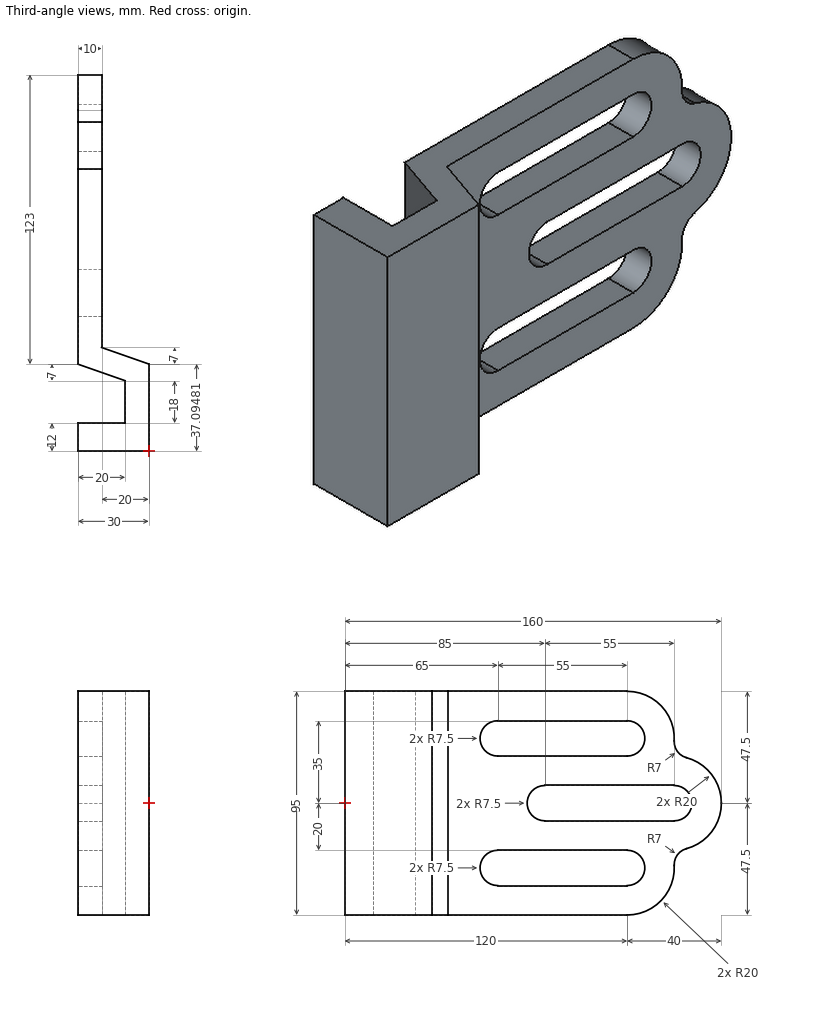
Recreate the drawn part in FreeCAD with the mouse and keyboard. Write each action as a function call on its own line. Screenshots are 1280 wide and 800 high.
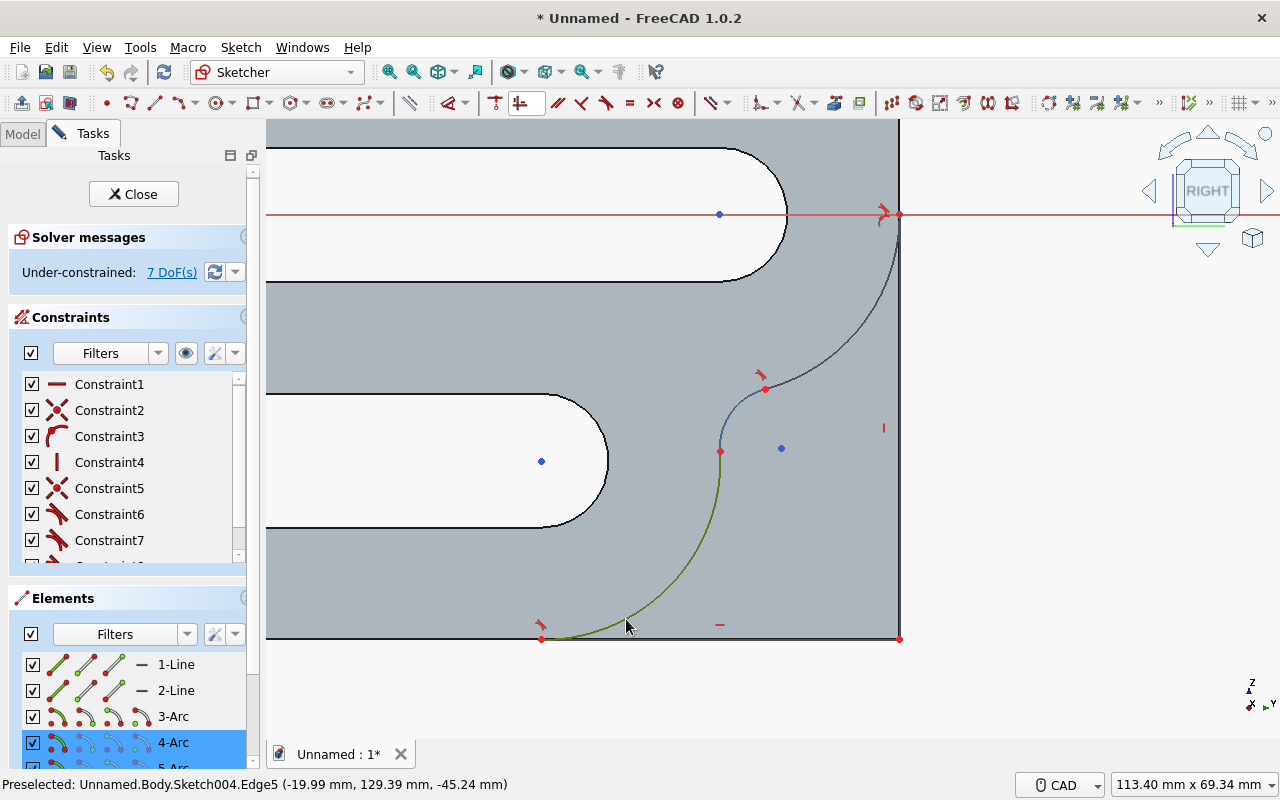
click(606, 104)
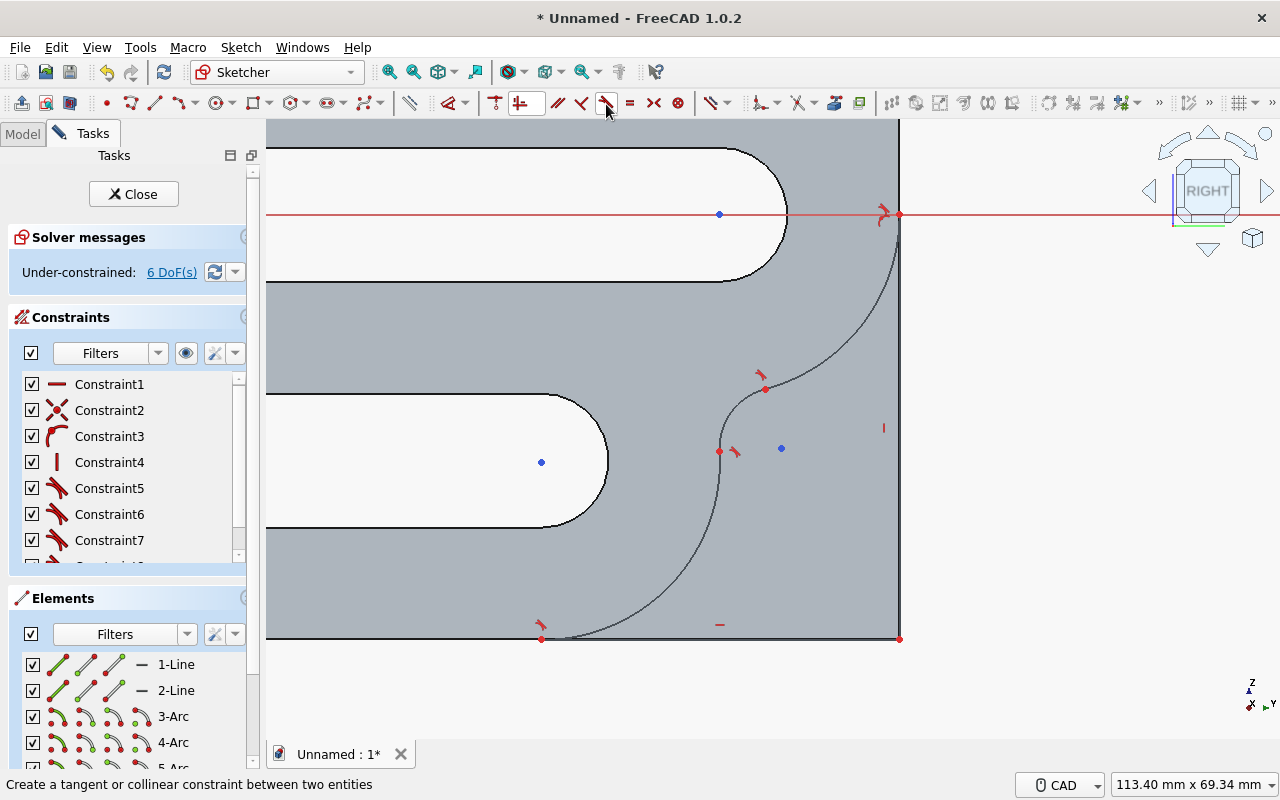
click(829, 358)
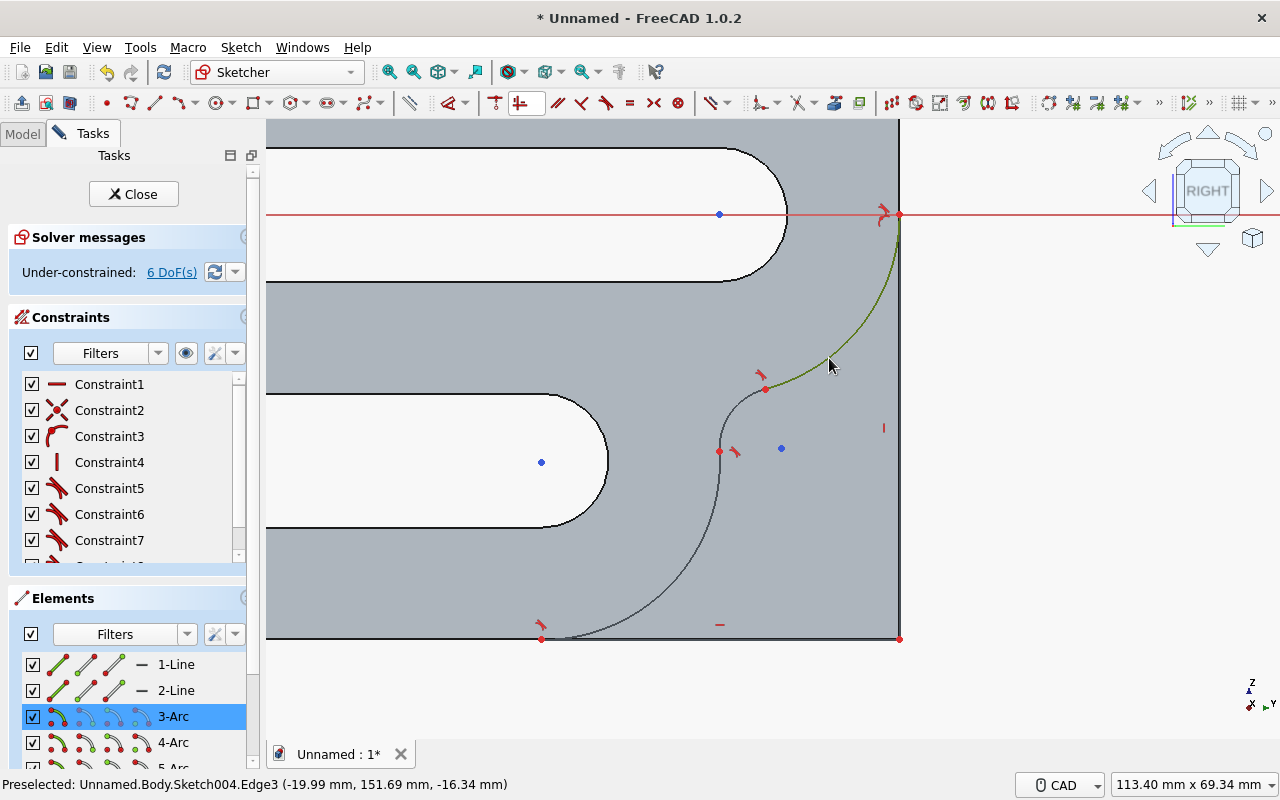
click(625, 619)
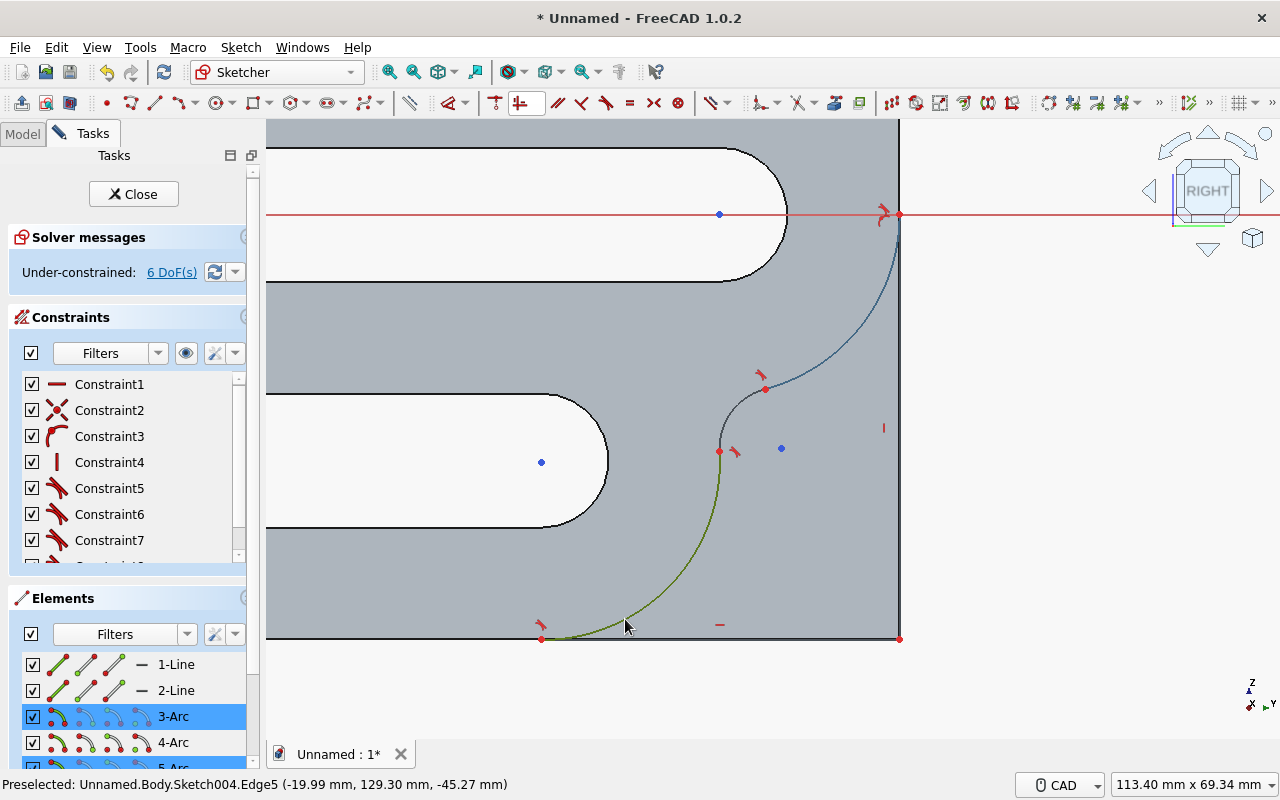
click(630, 104)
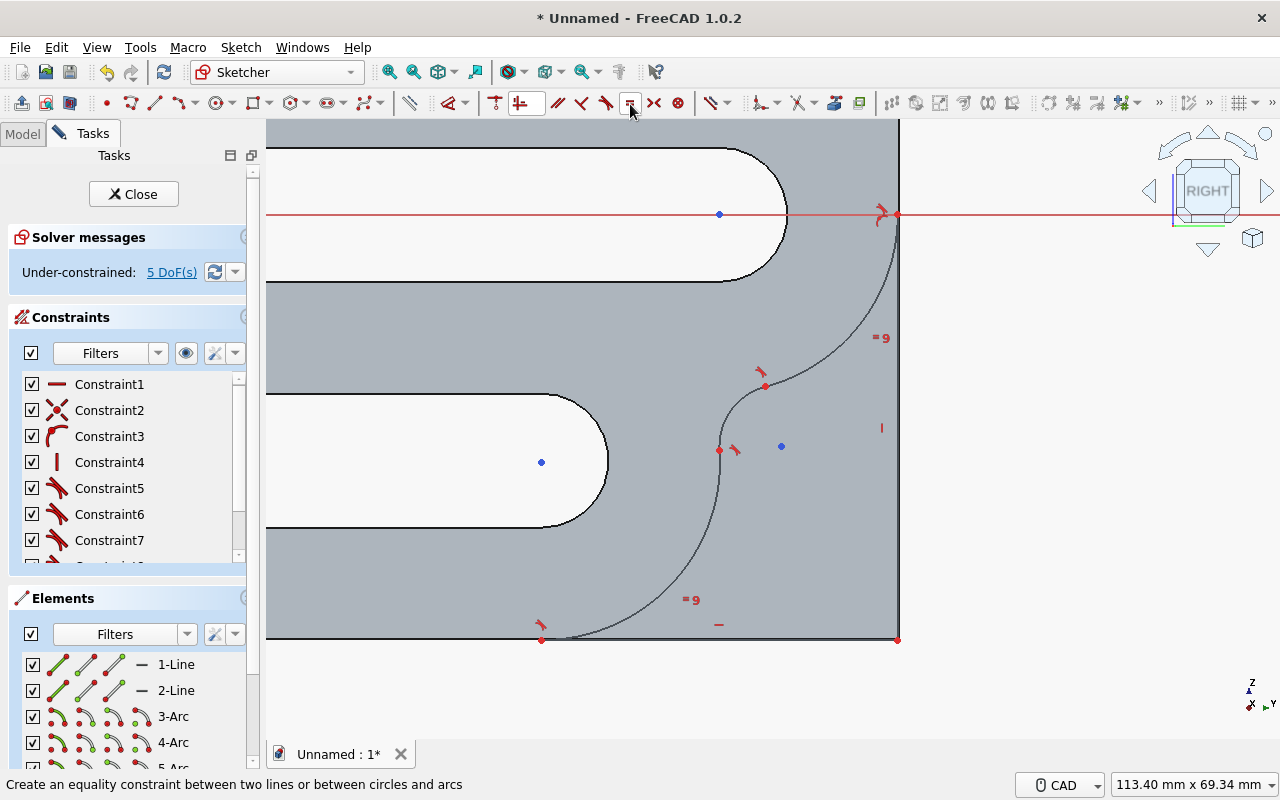
click(448, 104)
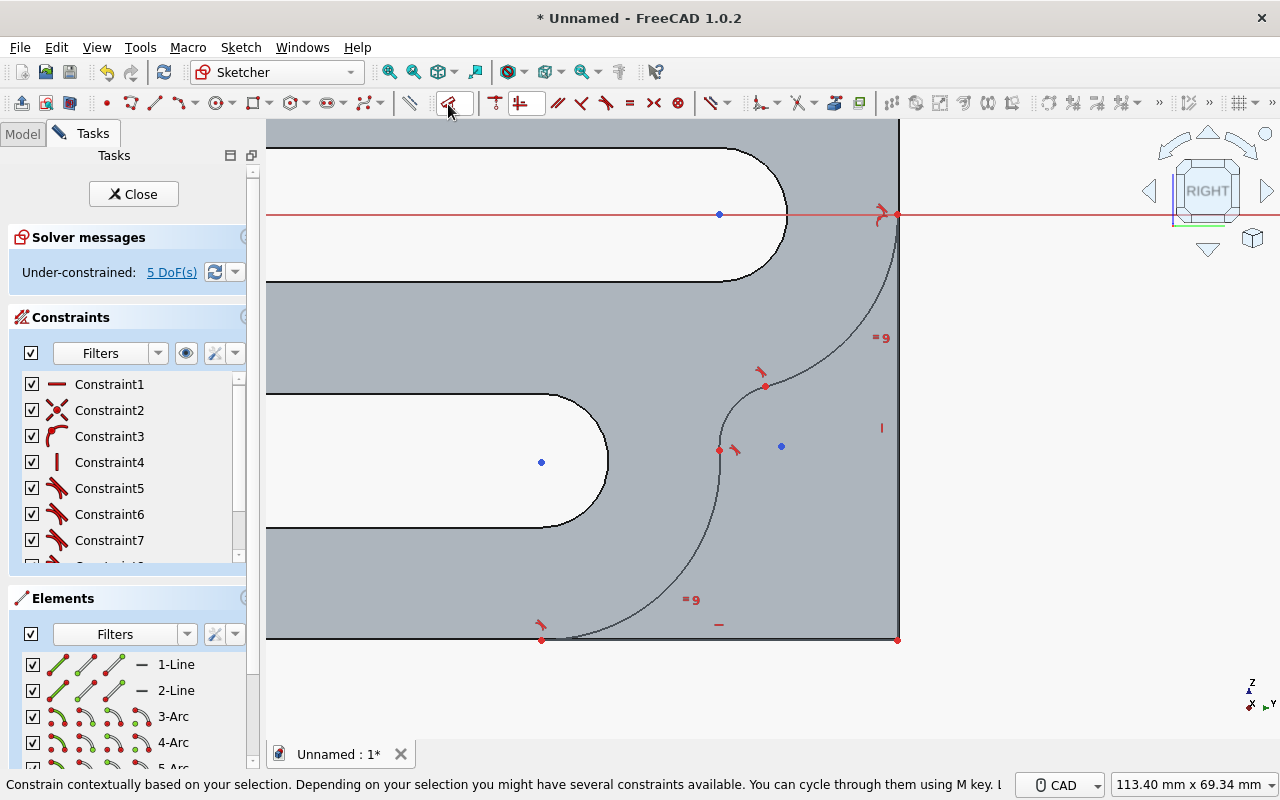
click(828, 356)
click(847, 381)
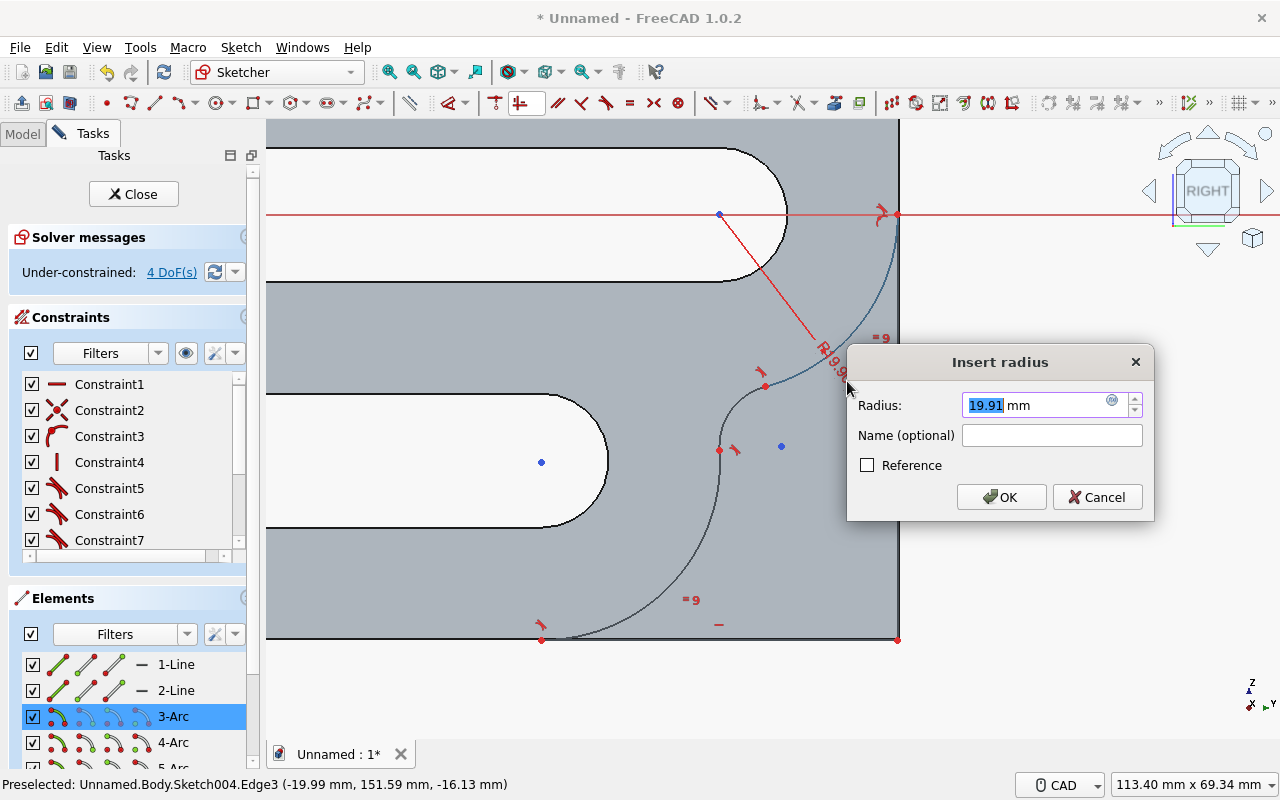
text(20)
key(Return)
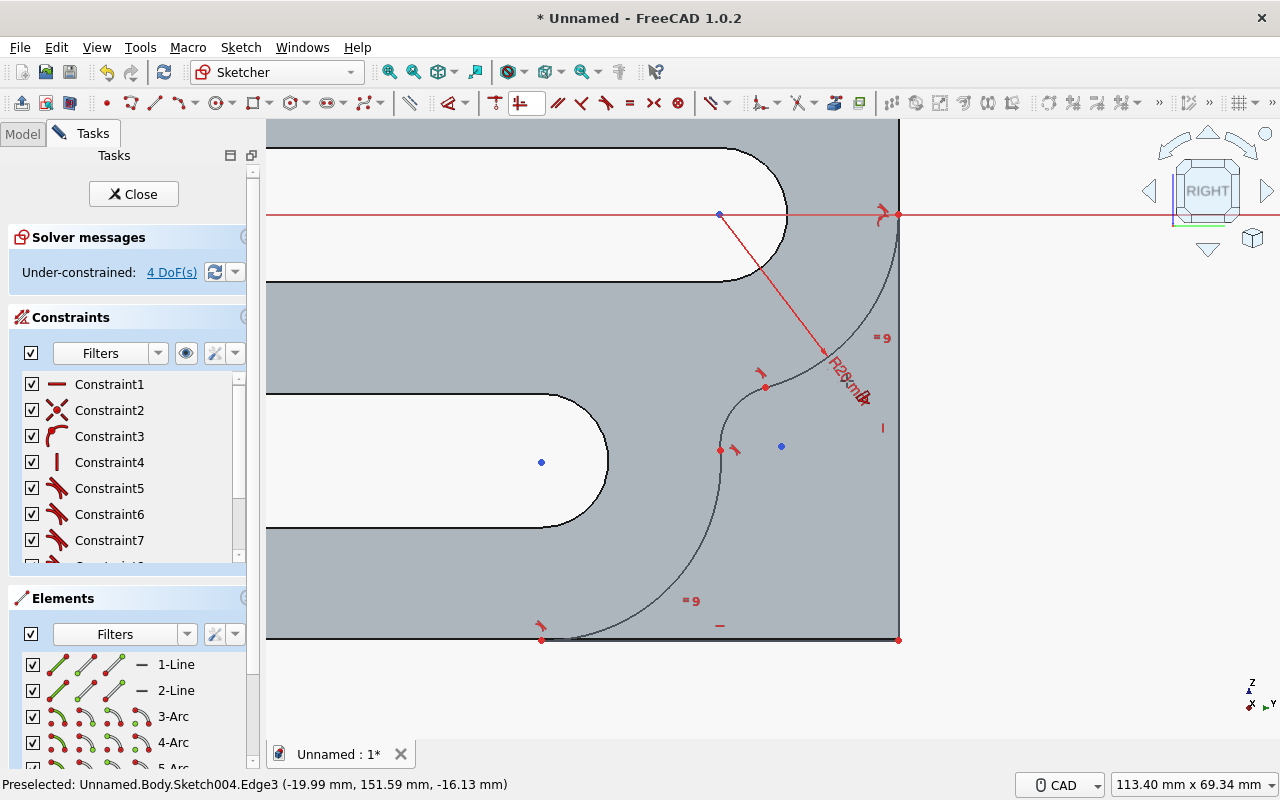
click(743, 399)
click(723, 374)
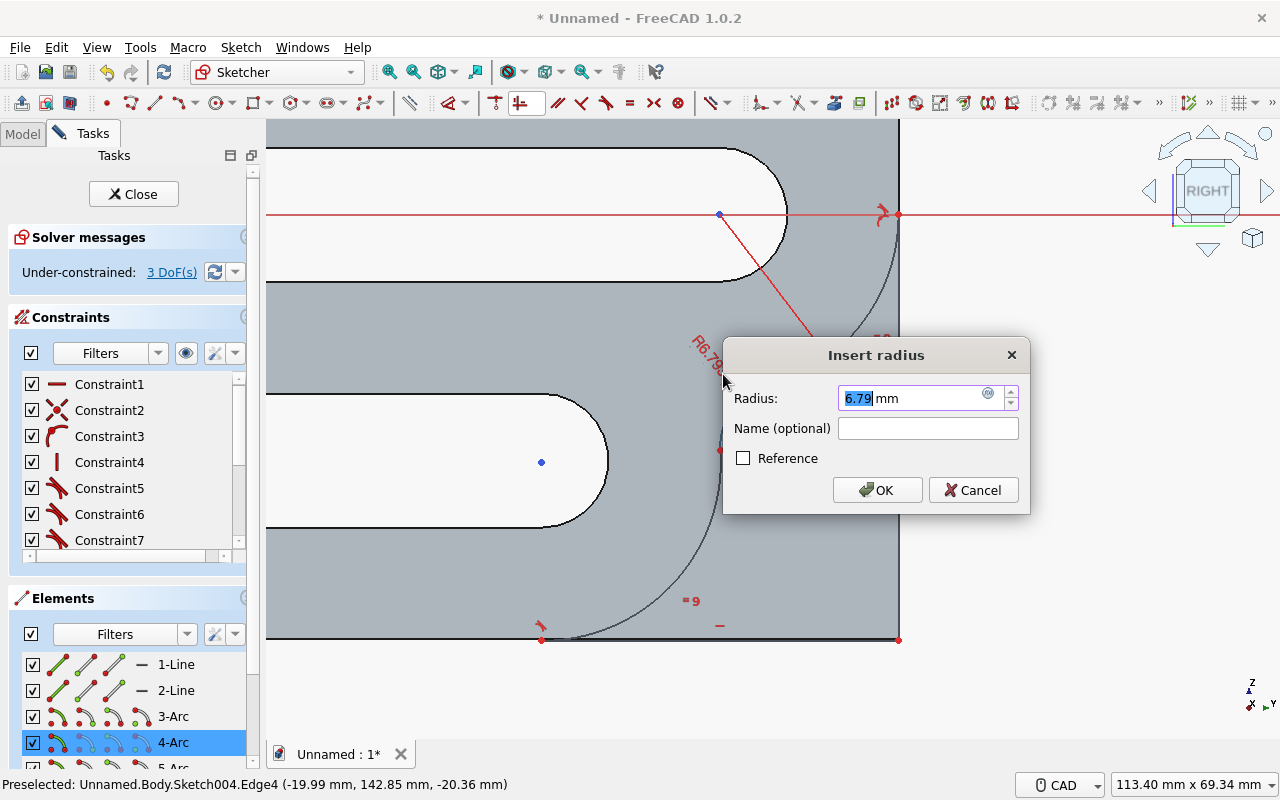
text(7)
key(Return)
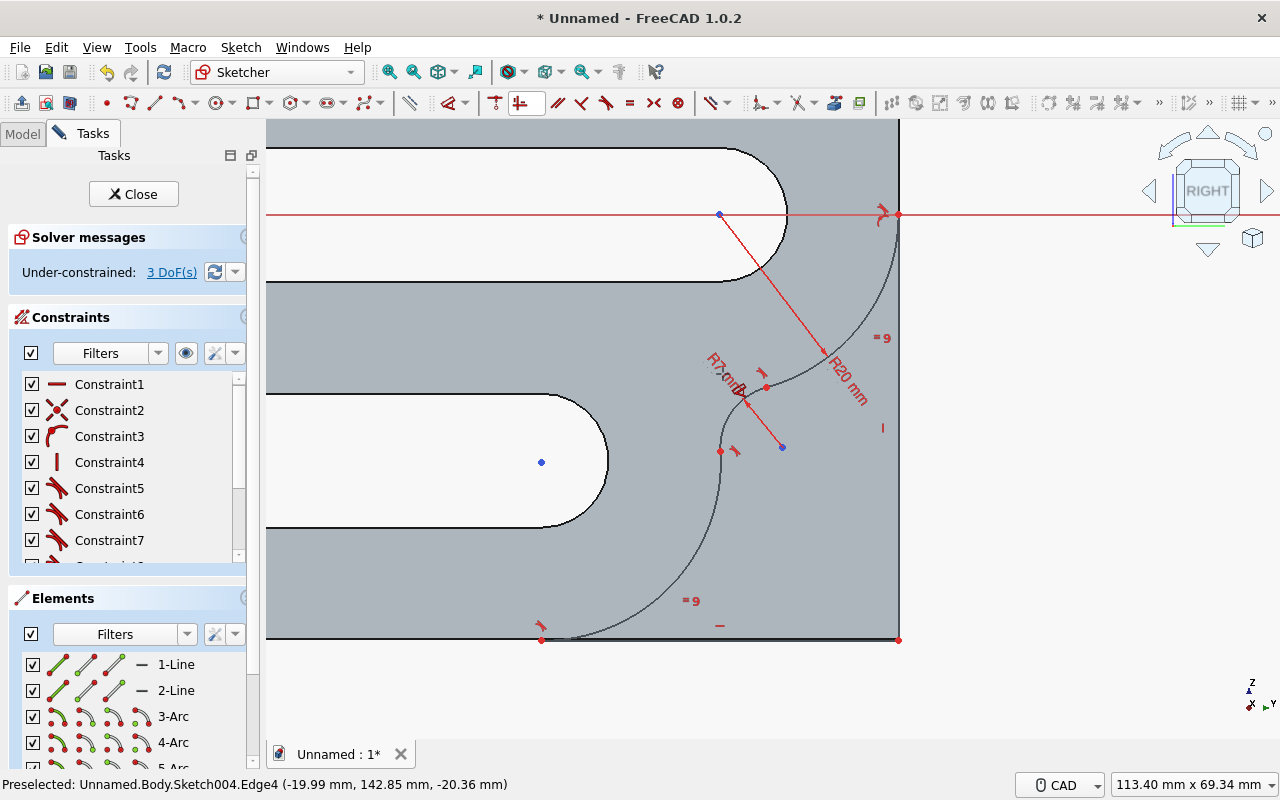
click(649, 641)
click(720, 675)